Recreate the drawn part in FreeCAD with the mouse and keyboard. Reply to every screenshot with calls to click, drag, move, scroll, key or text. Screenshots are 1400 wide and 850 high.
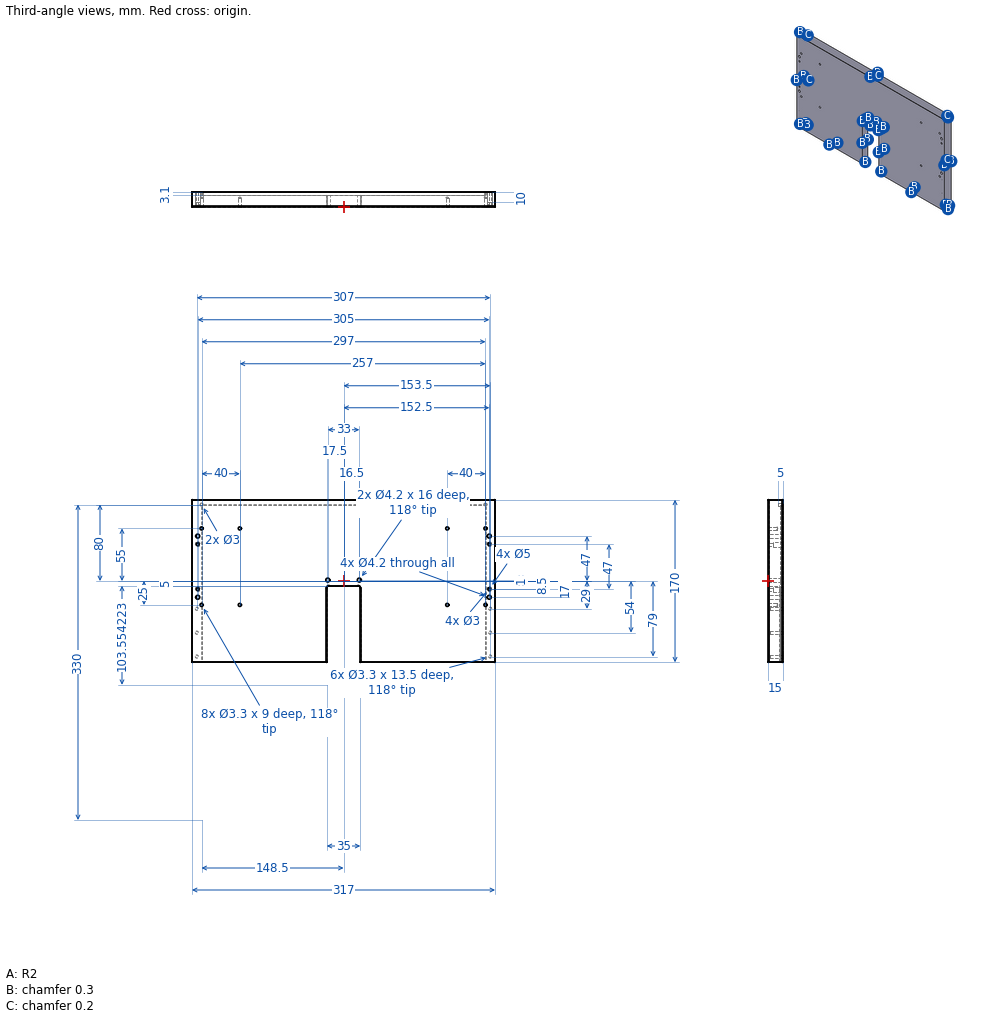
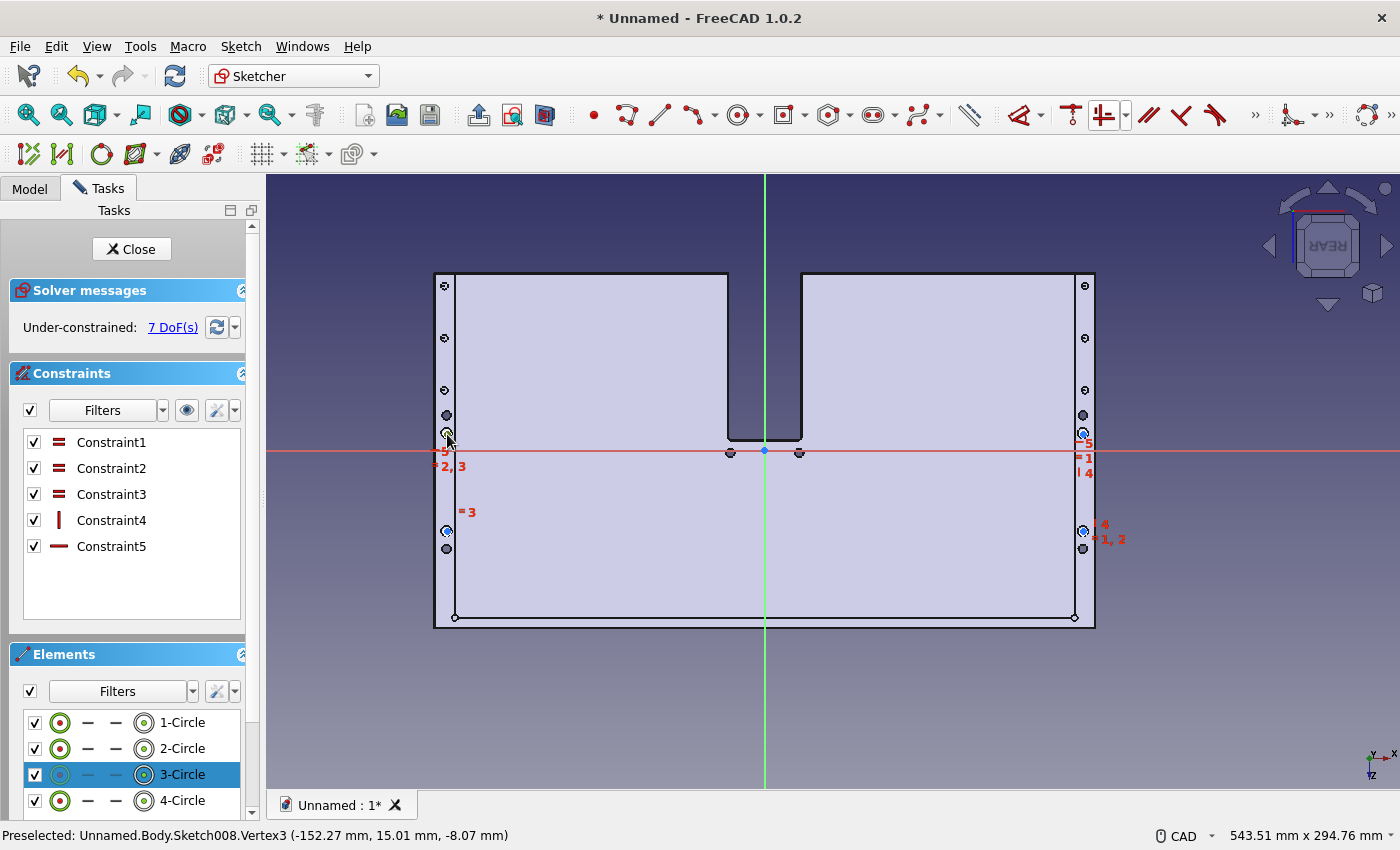
click(447, 532)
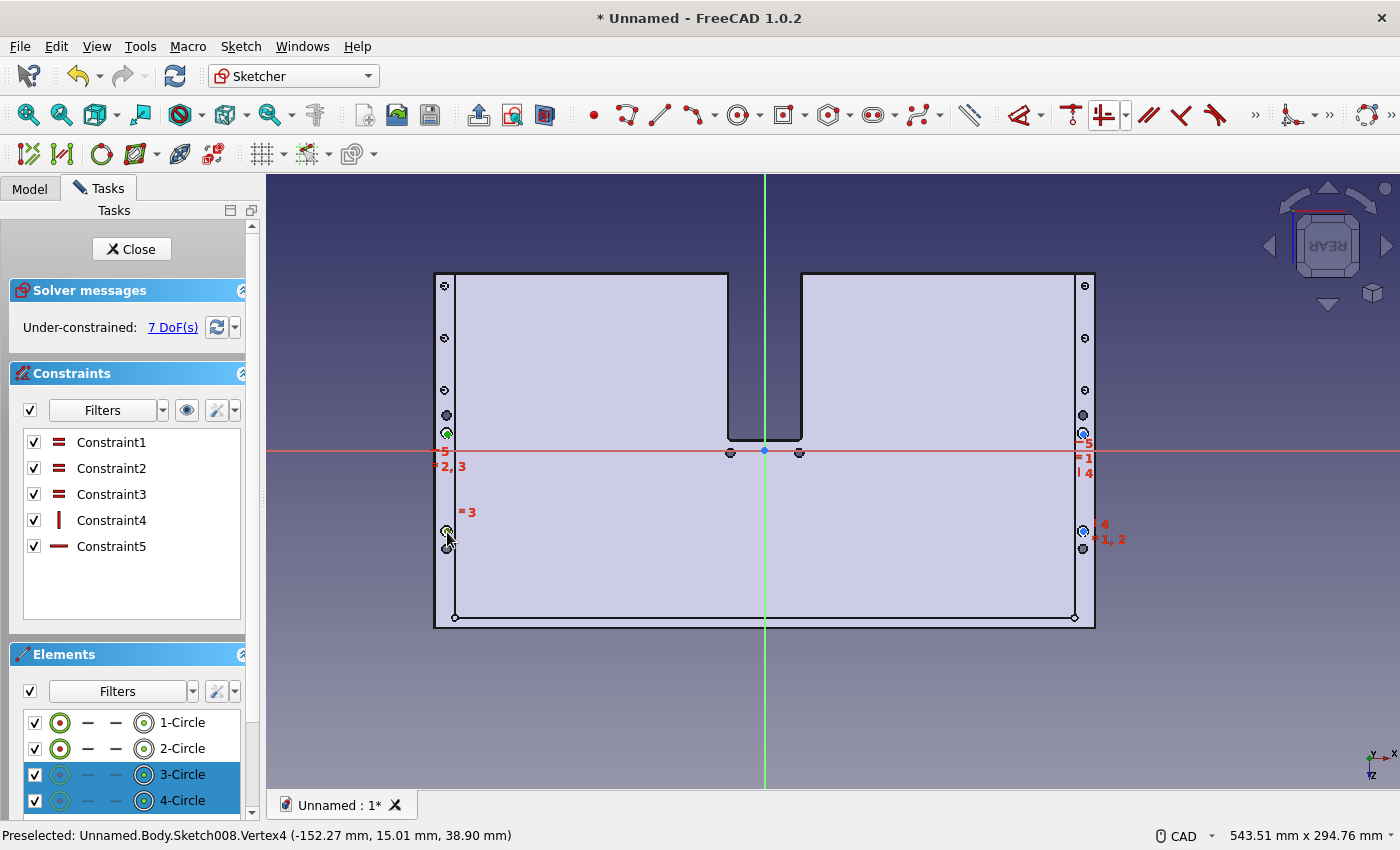
key(v)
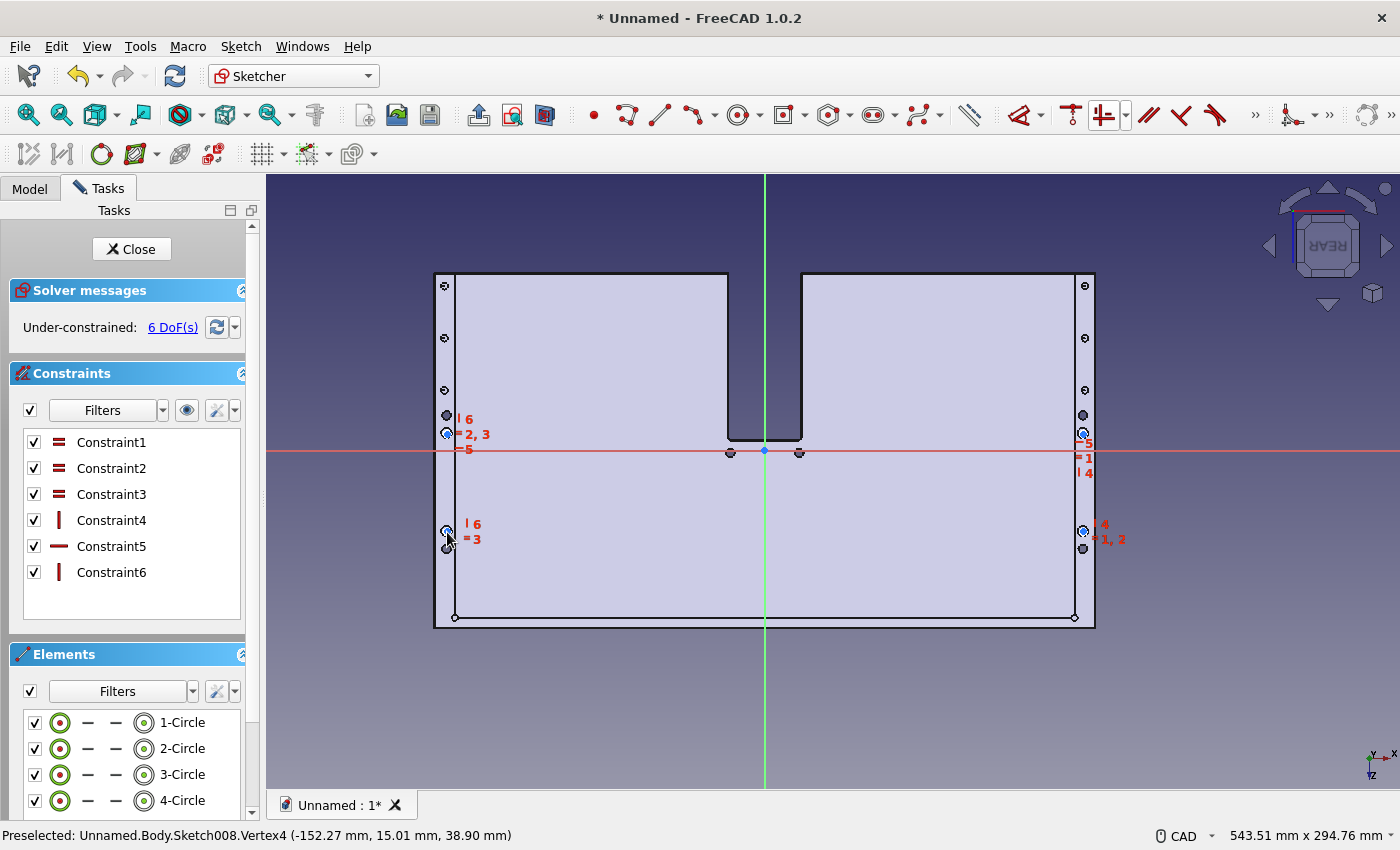
click(1083, 532)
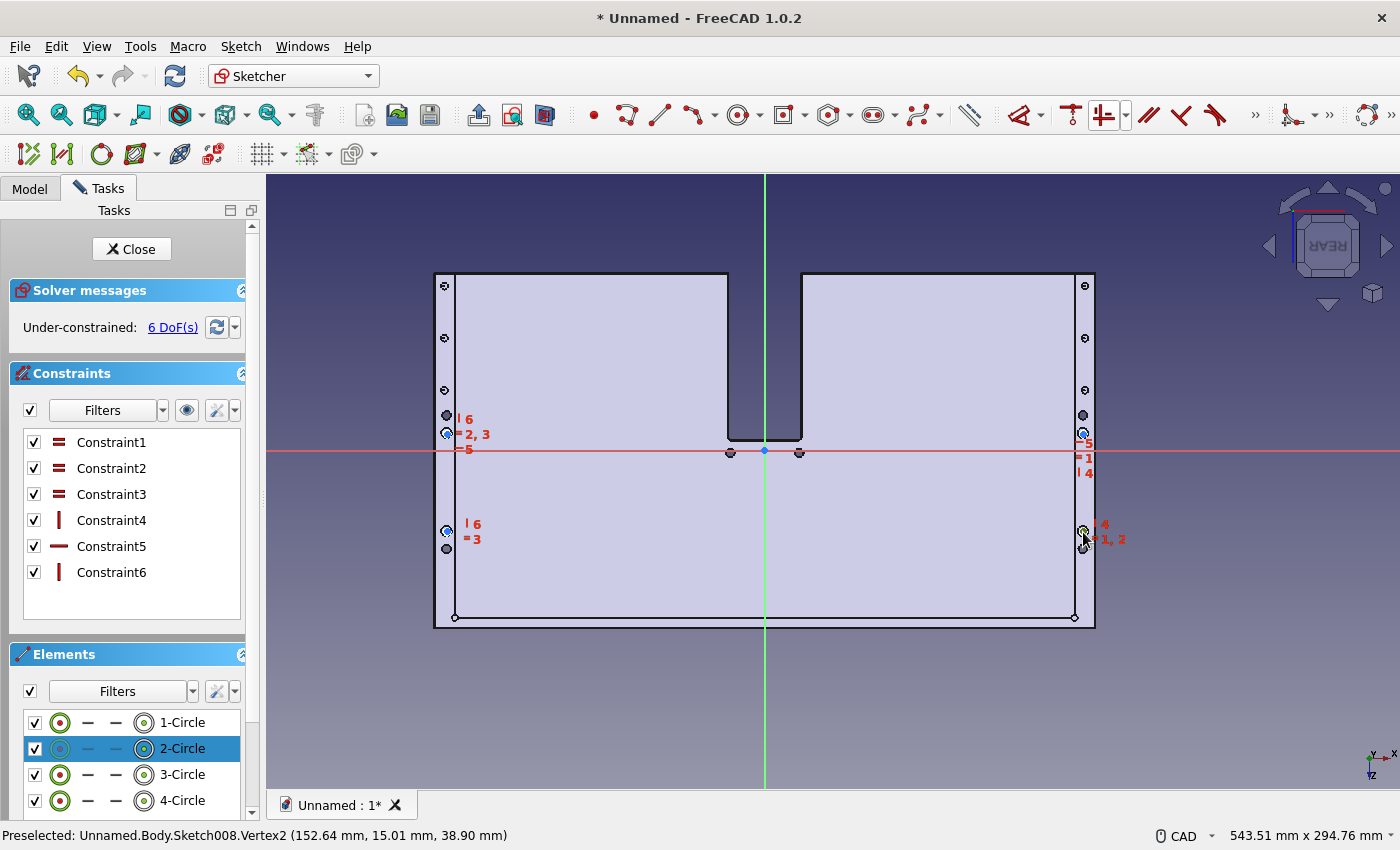
click(447, 532)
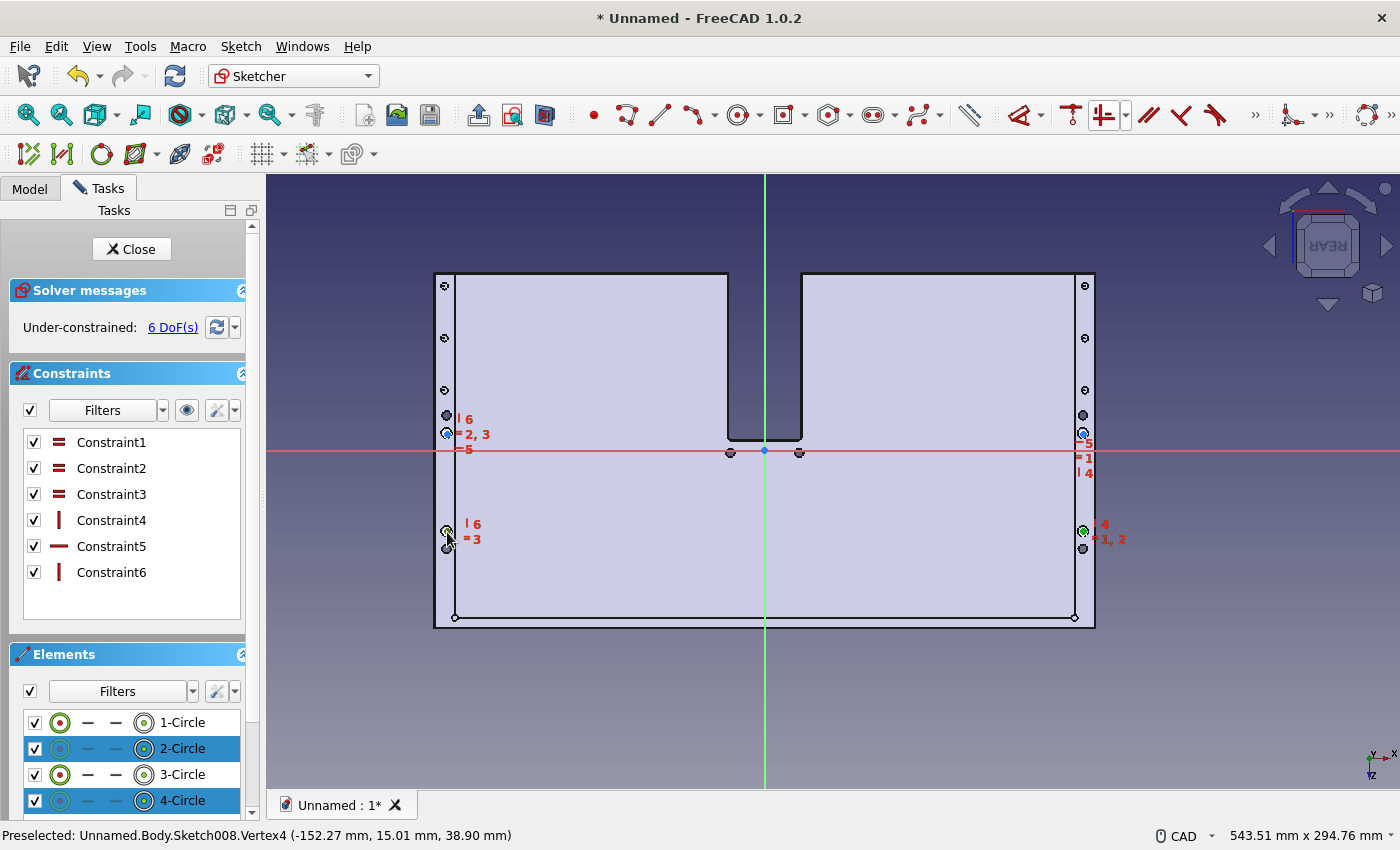
key(h)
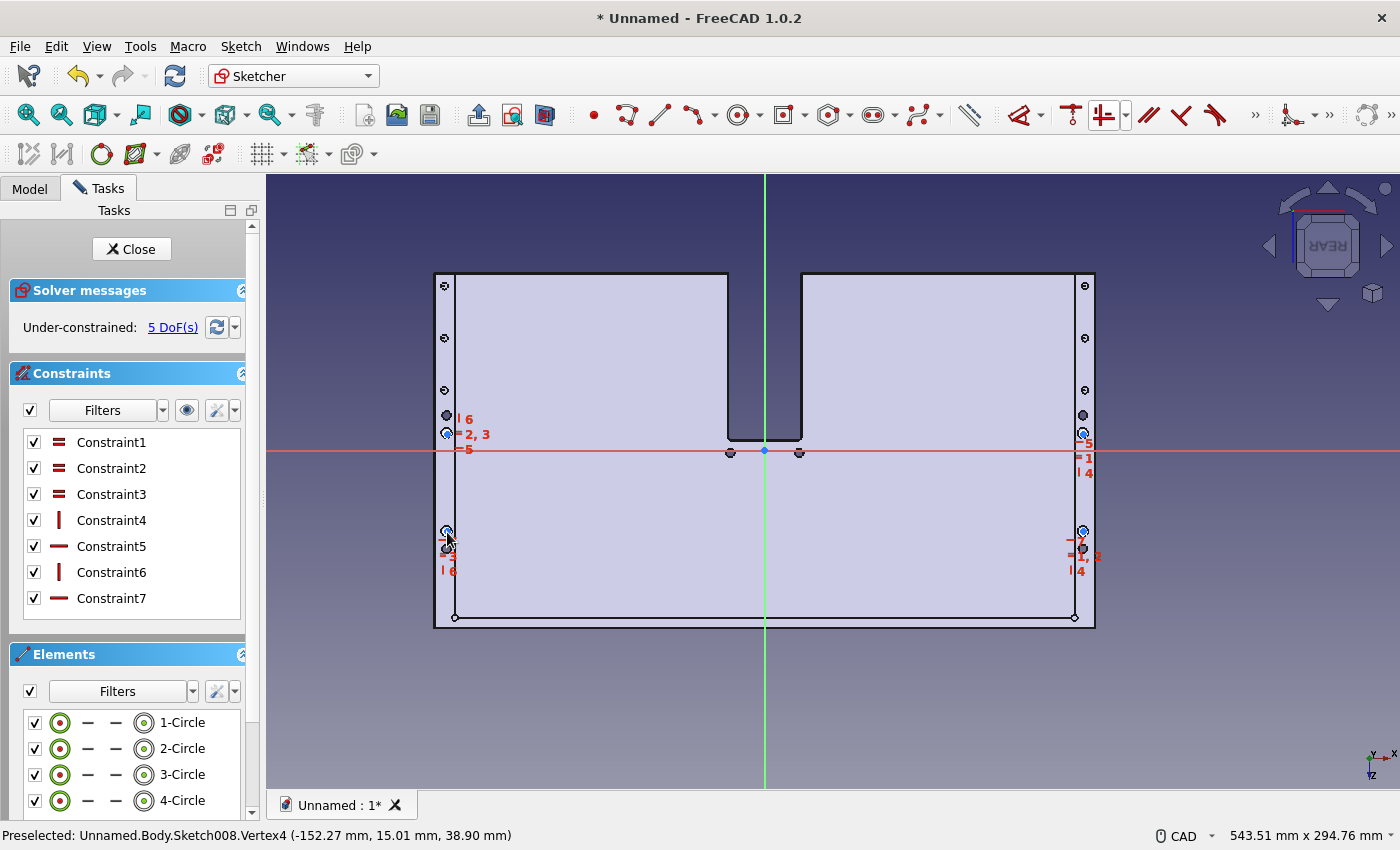
click(1018, 116)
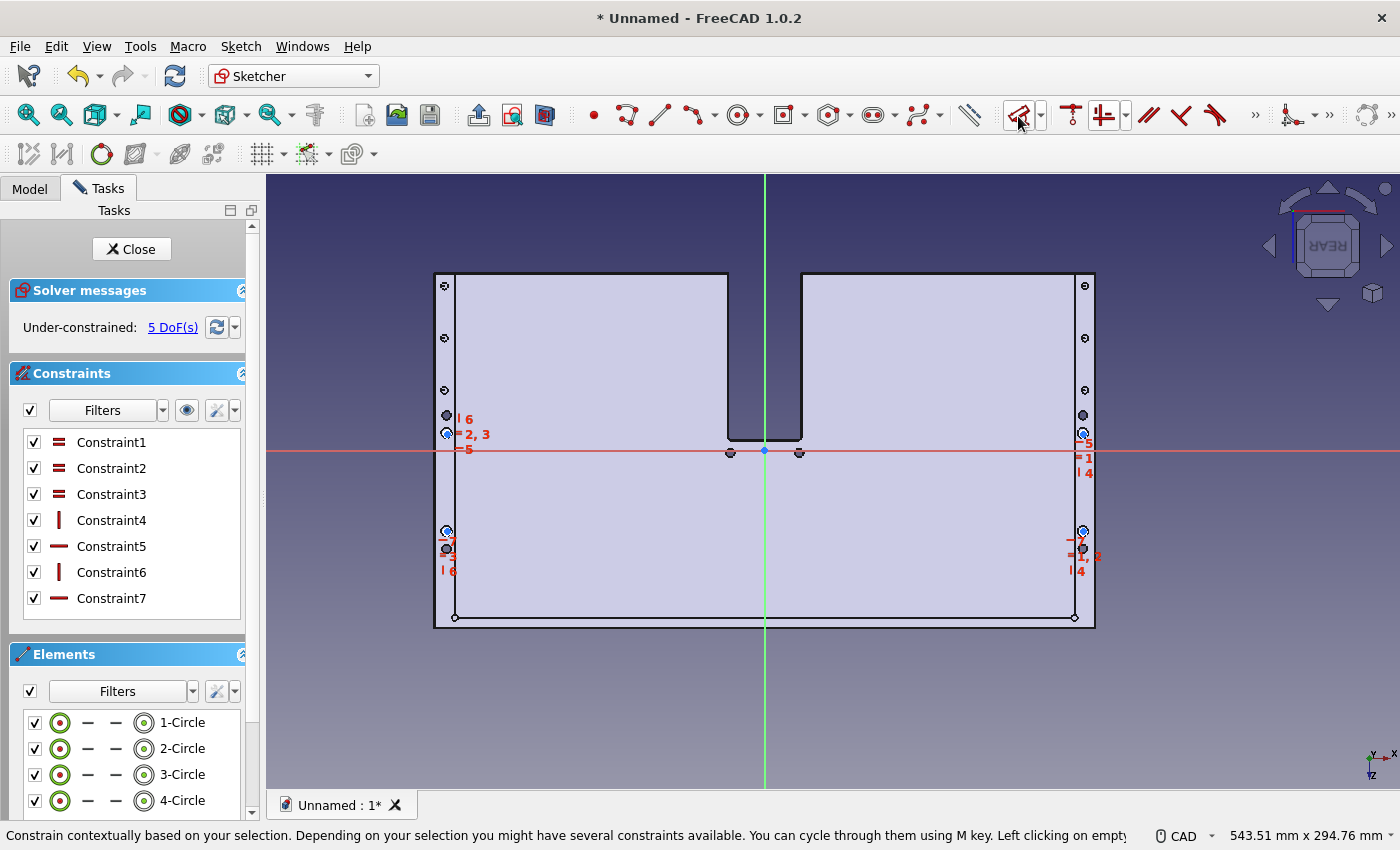
scroll(1081, 437, up, 10)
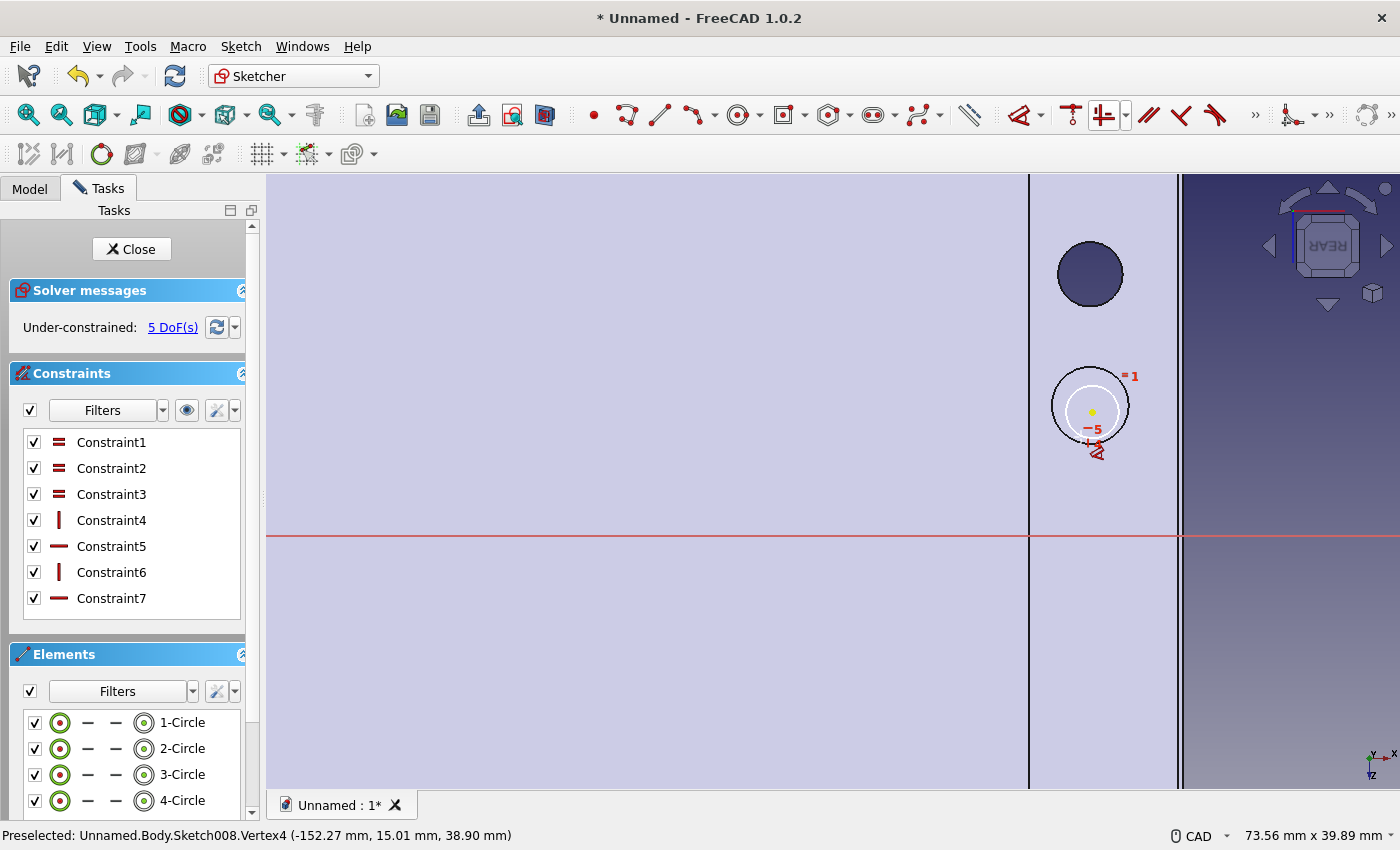
click(1074, 431)
click(1052, 454)